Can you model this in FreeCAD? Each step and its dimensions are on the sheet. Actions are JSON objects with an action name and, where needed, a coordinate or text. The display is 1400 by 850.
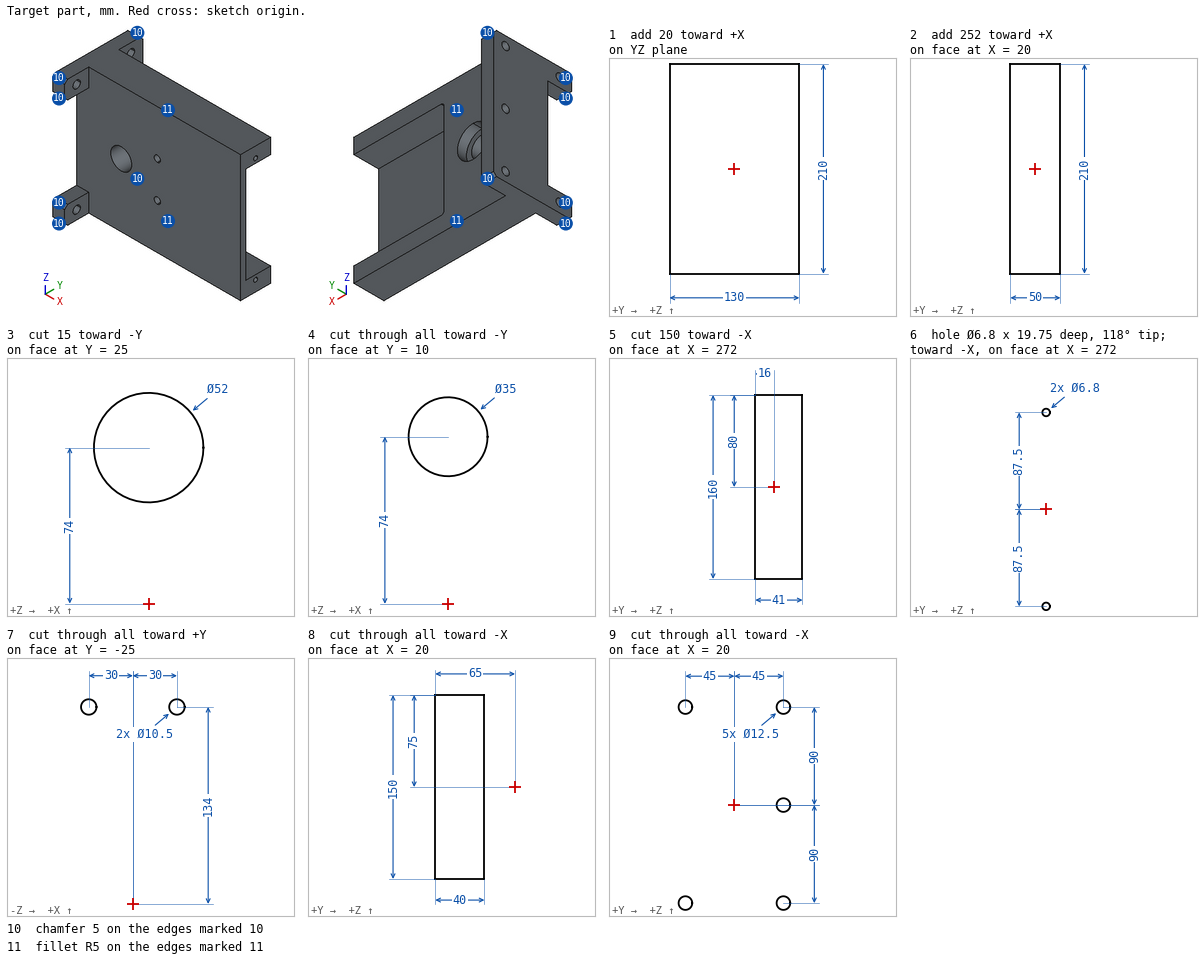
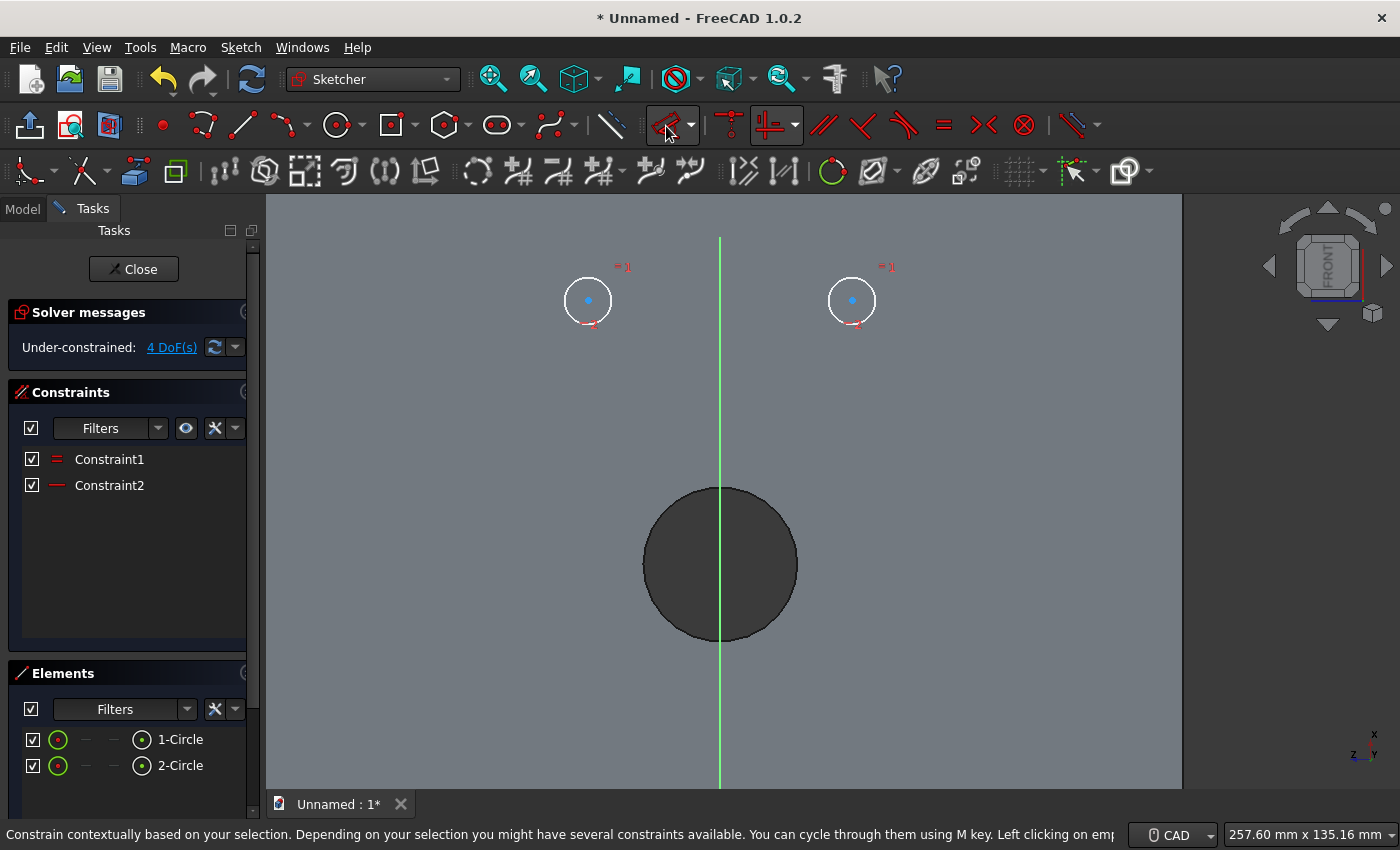
{"action": "left_click", "coordinate": [868, 284]}
{"action": "left_click", "coordinate": [890, 261]}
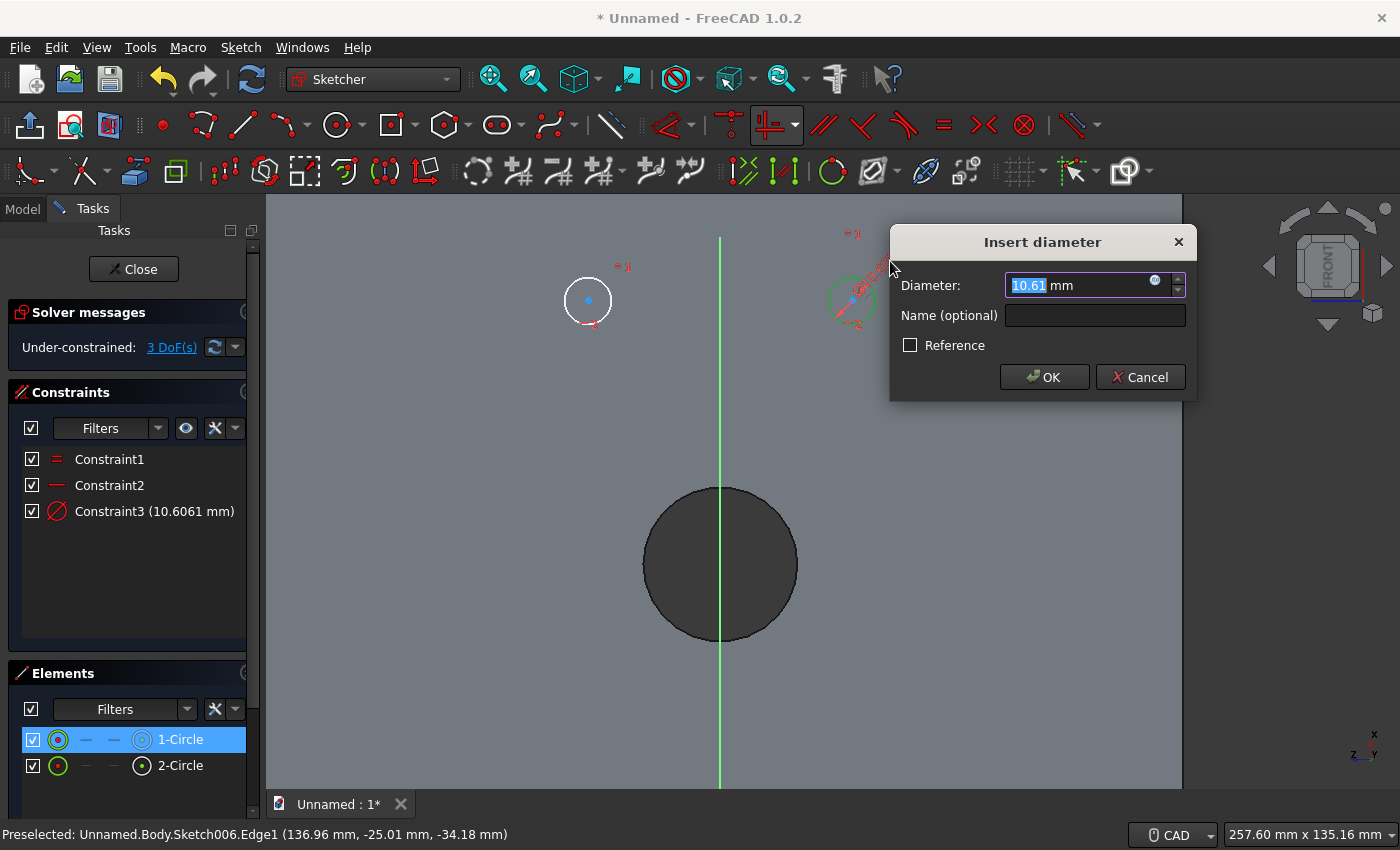
{"action": "type", "text": "10.5"}
{"action": "key", "text": "Return"}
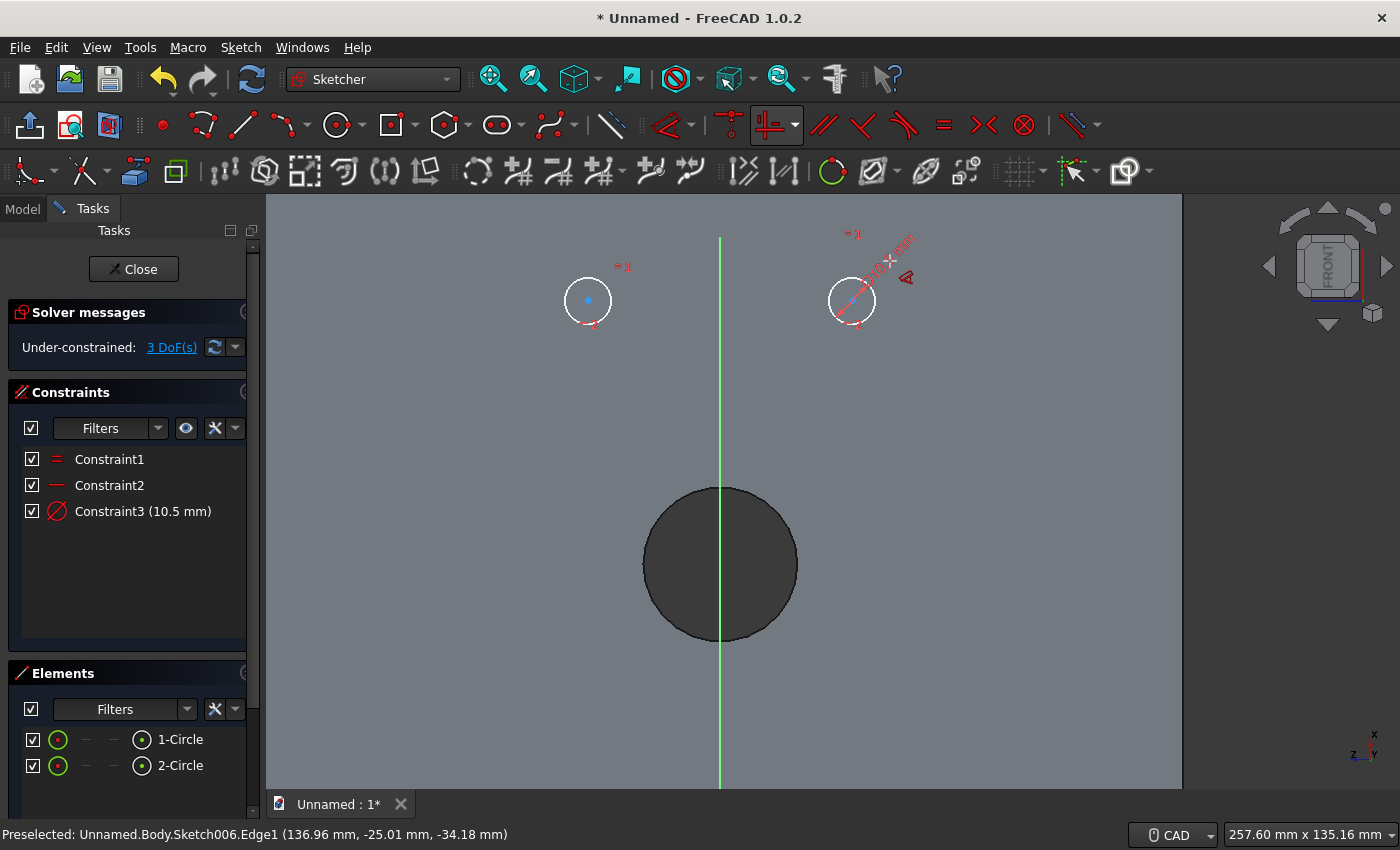
{"action": "left_click", "coordinate": [852, 301]}
{"action": "left_click", "coordinate": [786, 267]}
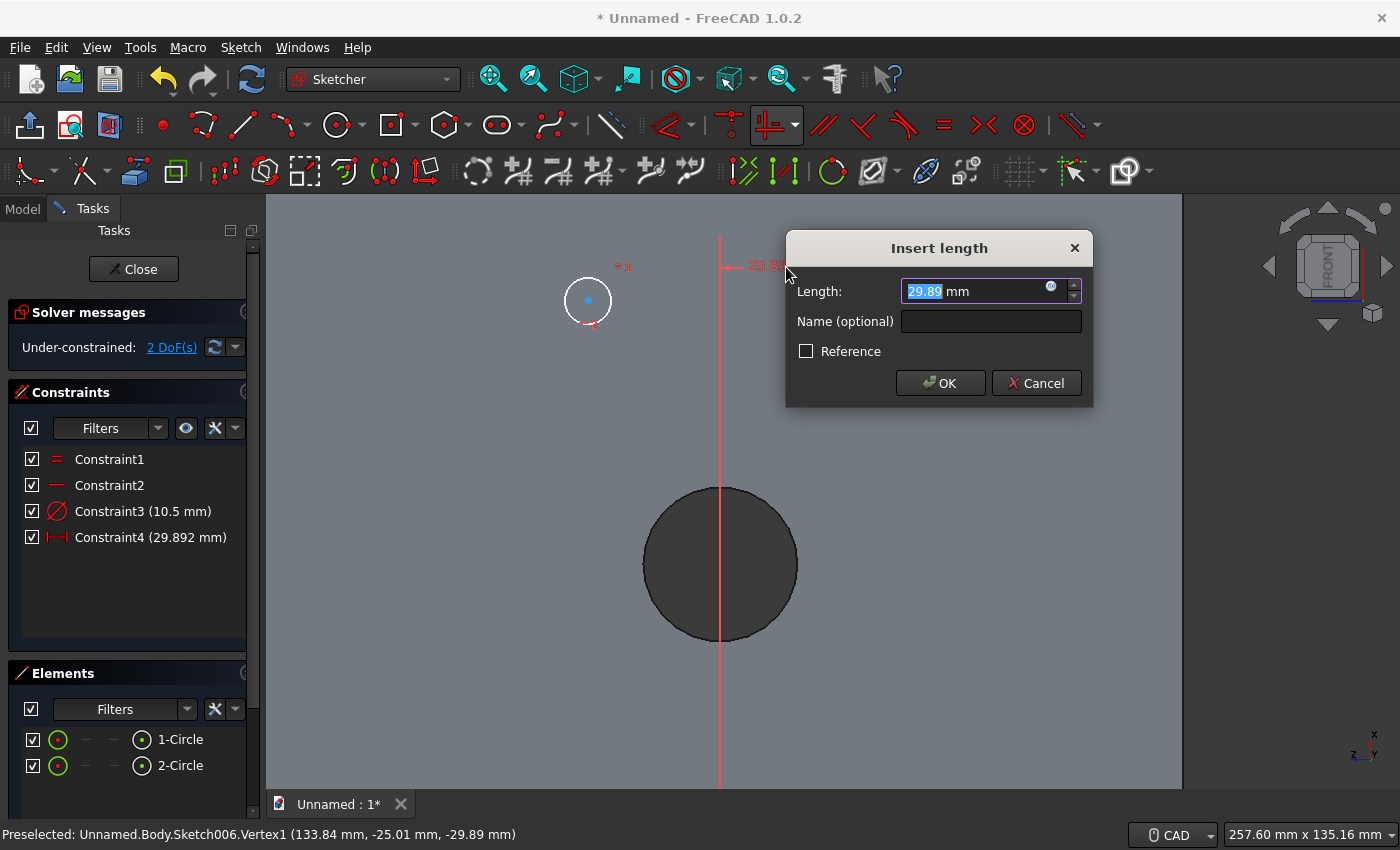
{"action": "type", "text": "30"}
{"action": "key", "text": "Return"}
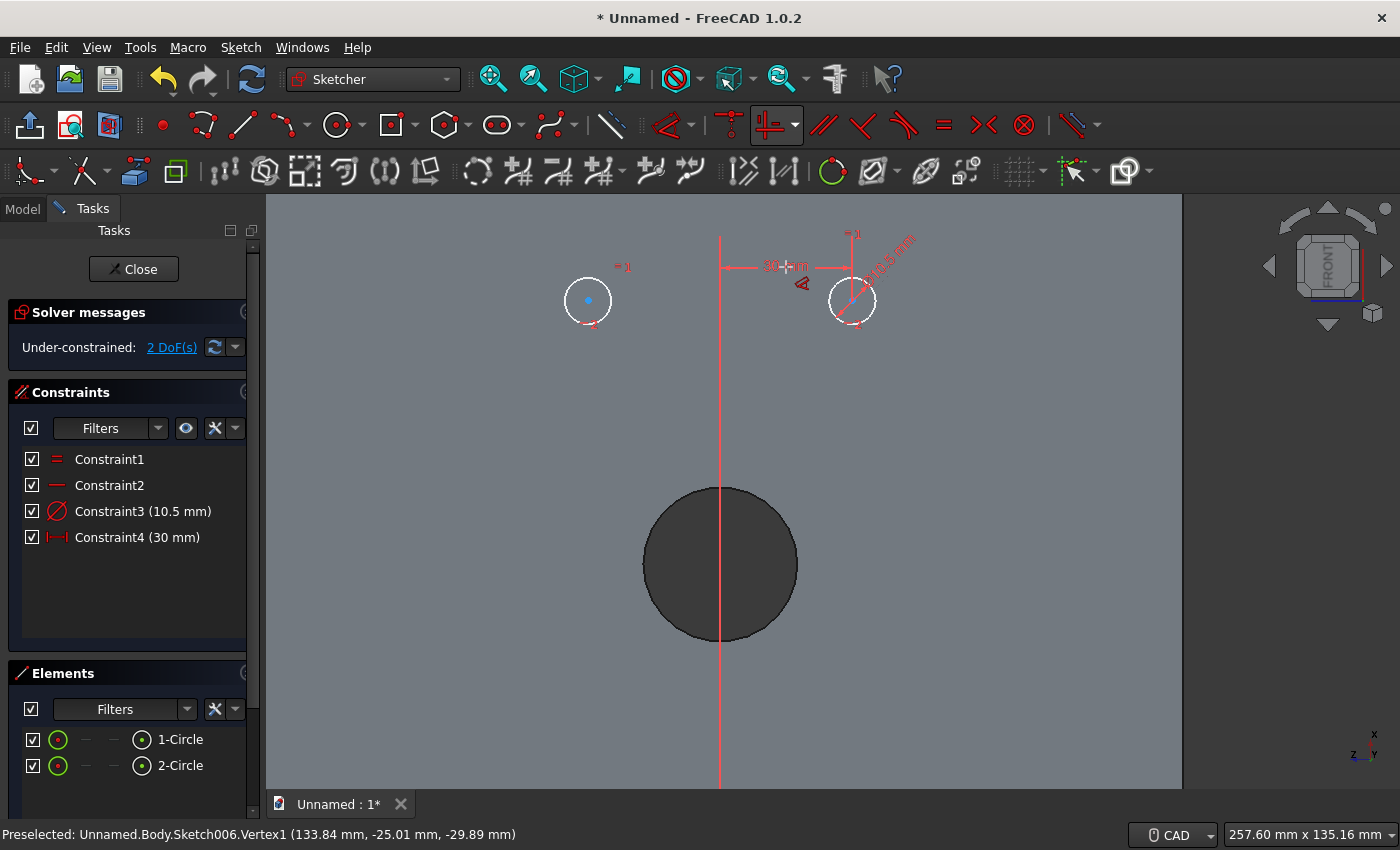
{"action": "left_click", "coordinate": [588, 301]}
{"action": "left_click", "coordinate": [654, 267]}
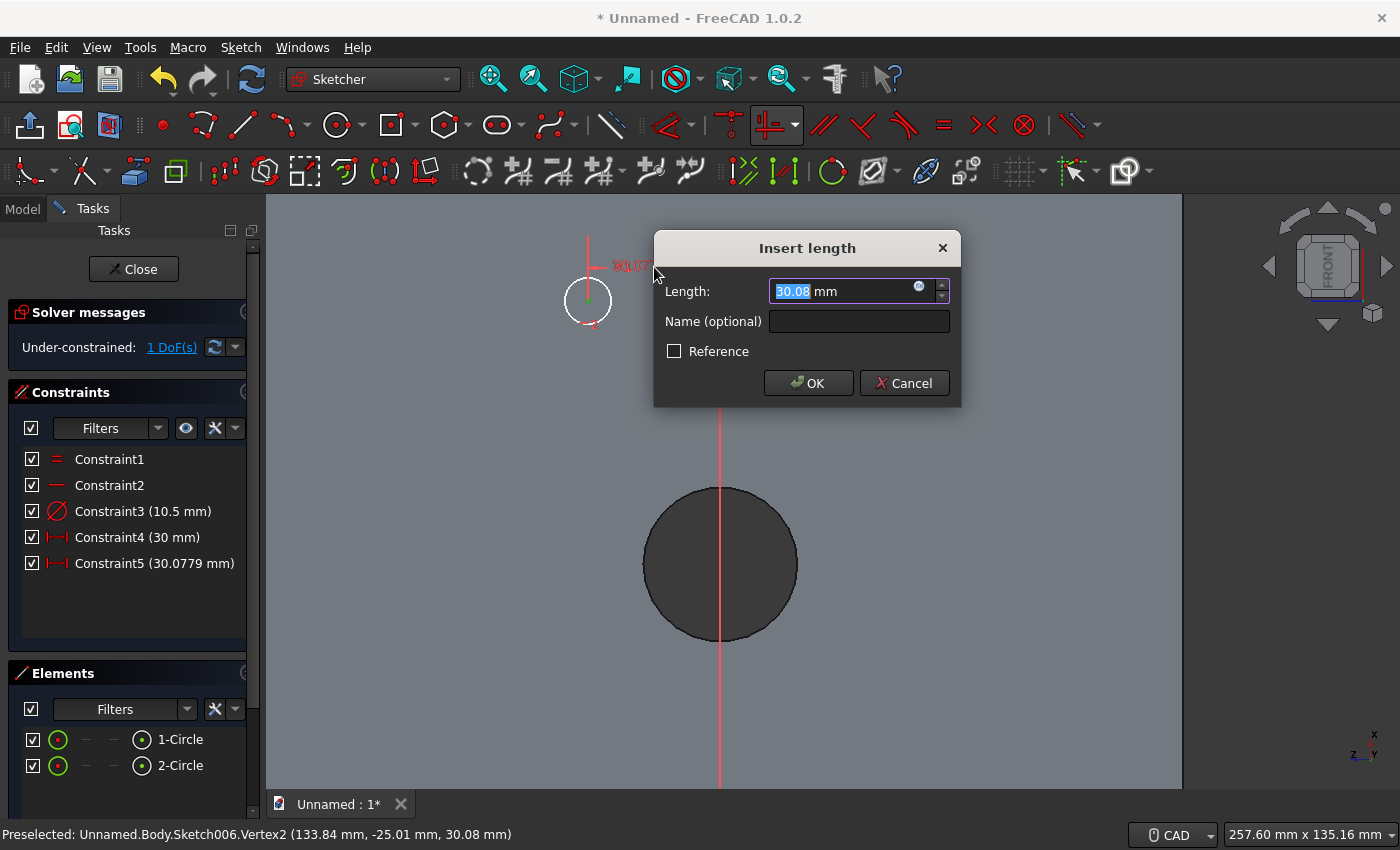
{"action": "type", "text": "30"}
{"action": "key", "text": "Return"}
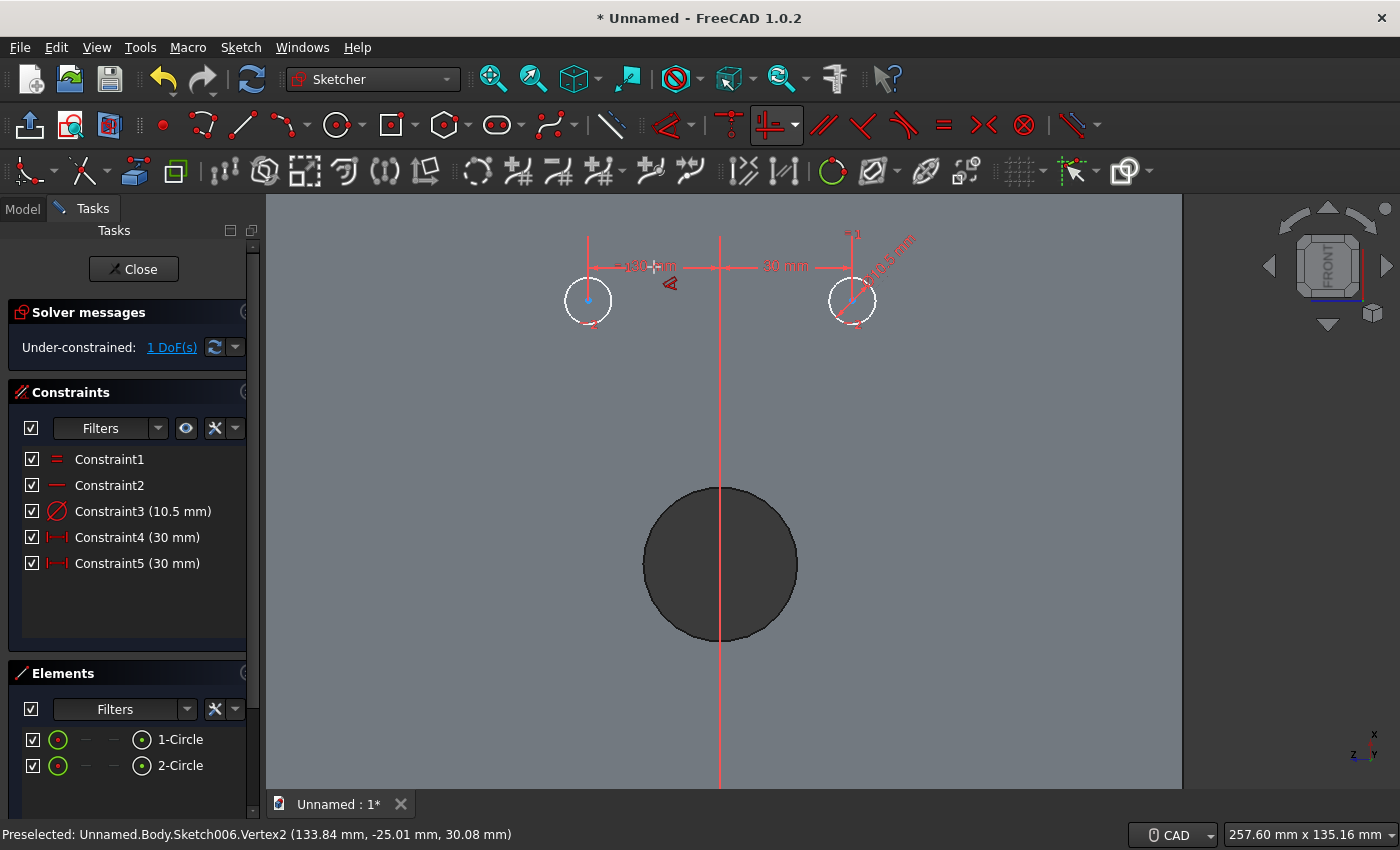
{"action": "left_click", "coordinate": [852, 301]}
{"action": "left_click", "coordinate": [886, 531]}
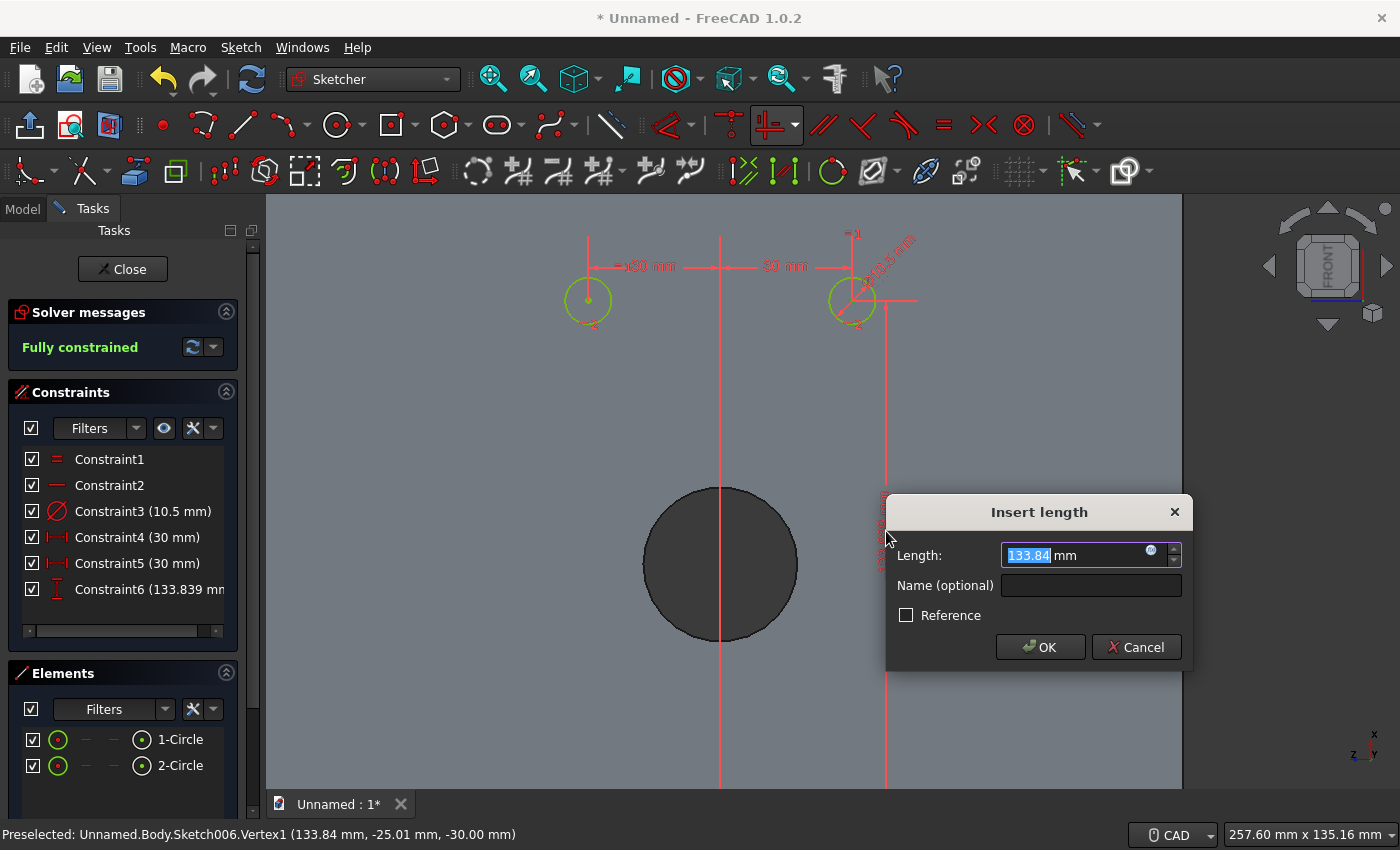
{"action": "type", "text": "134"}
{"action": "key", "text": "Return"}
{"action": "key", "text": "Escape"}